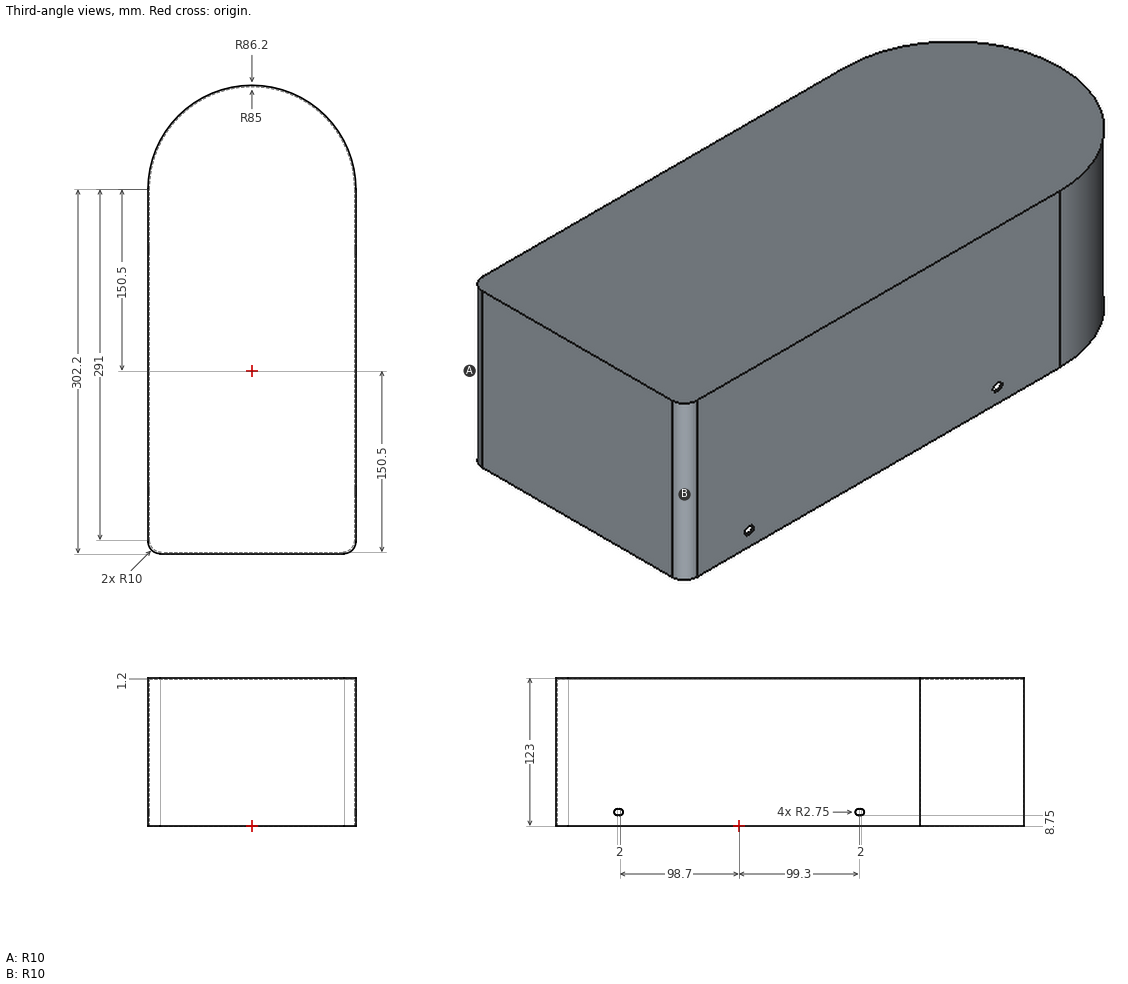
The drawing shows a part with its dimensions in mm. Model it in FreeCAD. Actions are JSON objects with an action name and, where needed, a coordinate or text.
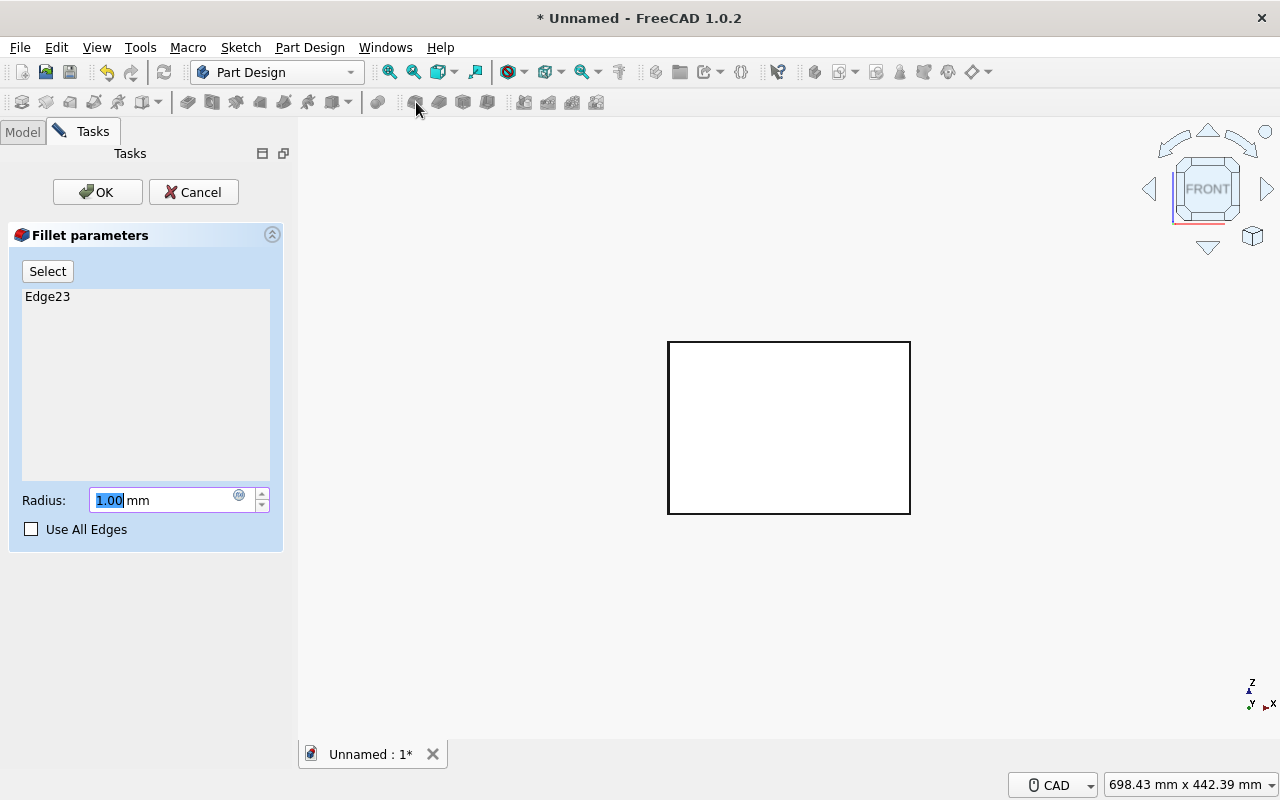
{"action": "type", "text": "10"}
{"action": "key", "text": "Tab"}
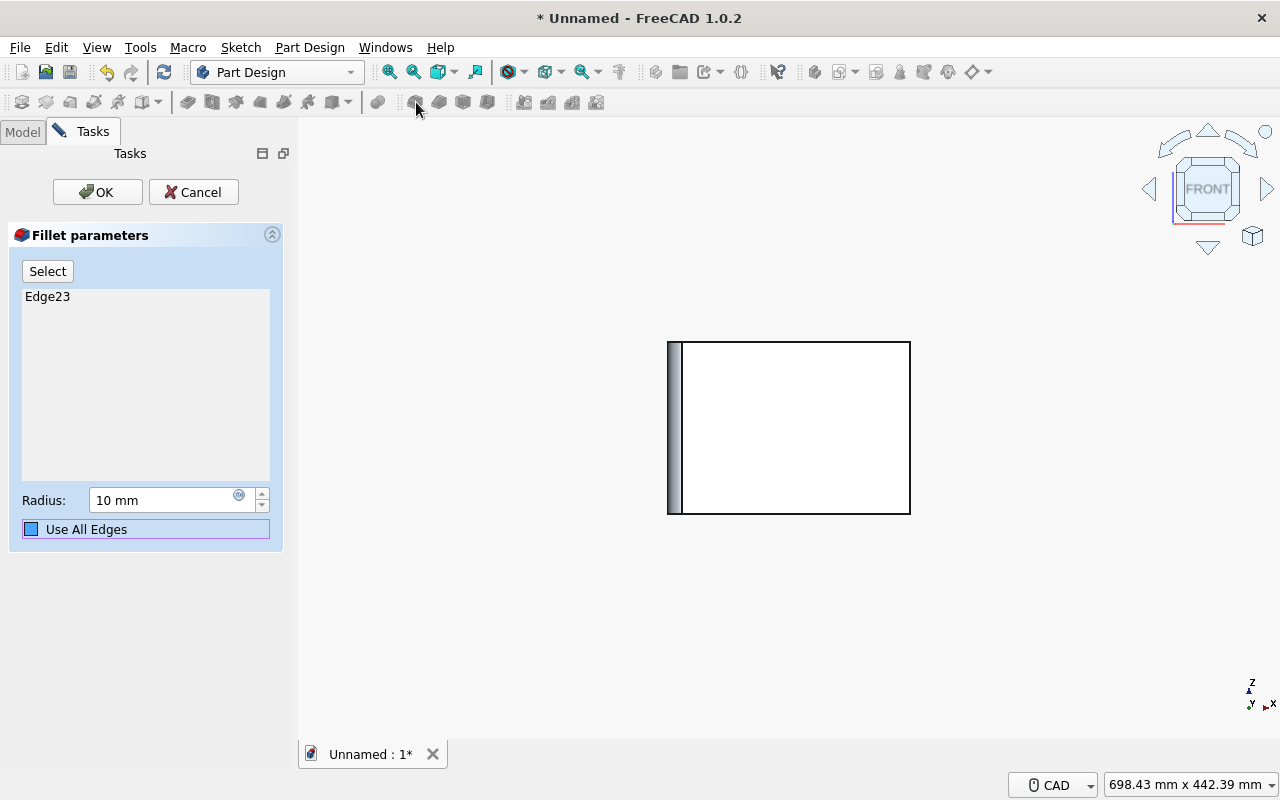
{"action": "left_click", "coordinate": [98, 192]}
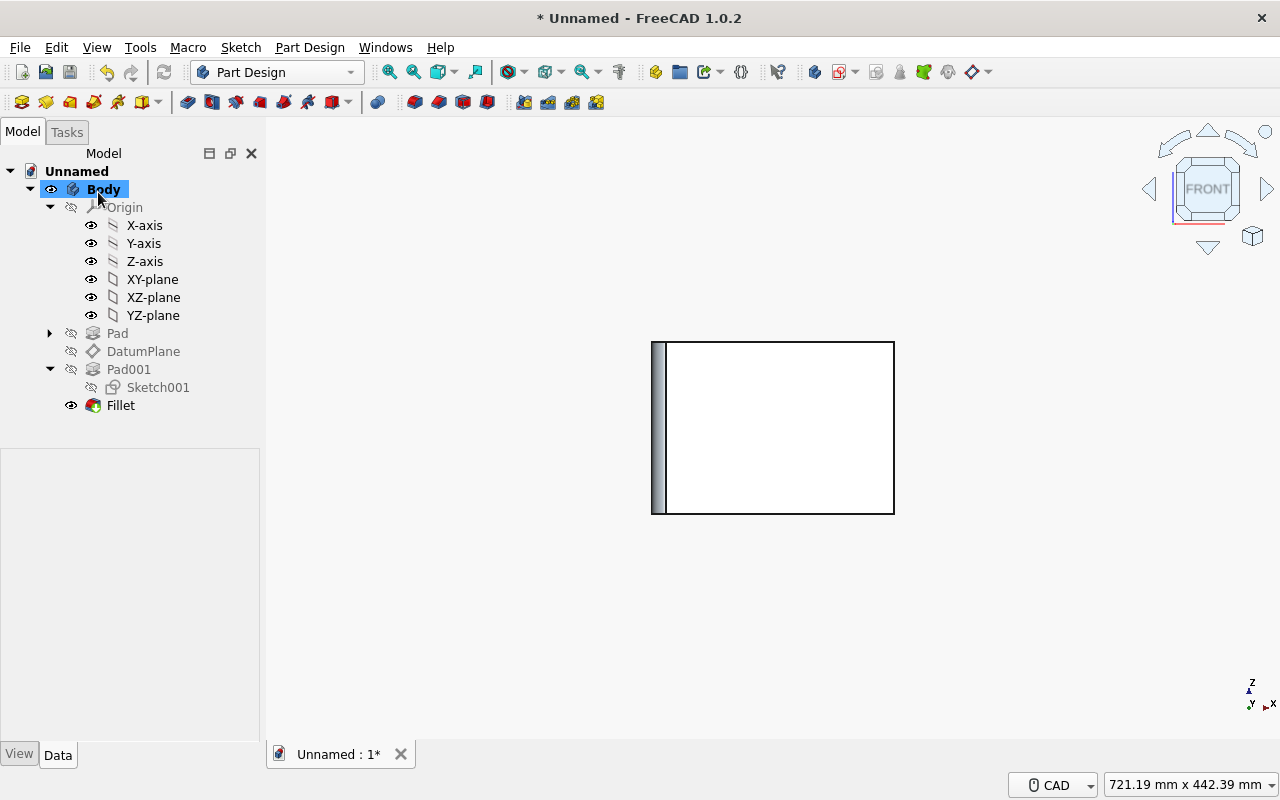
{"action": "key", "text": "v f"}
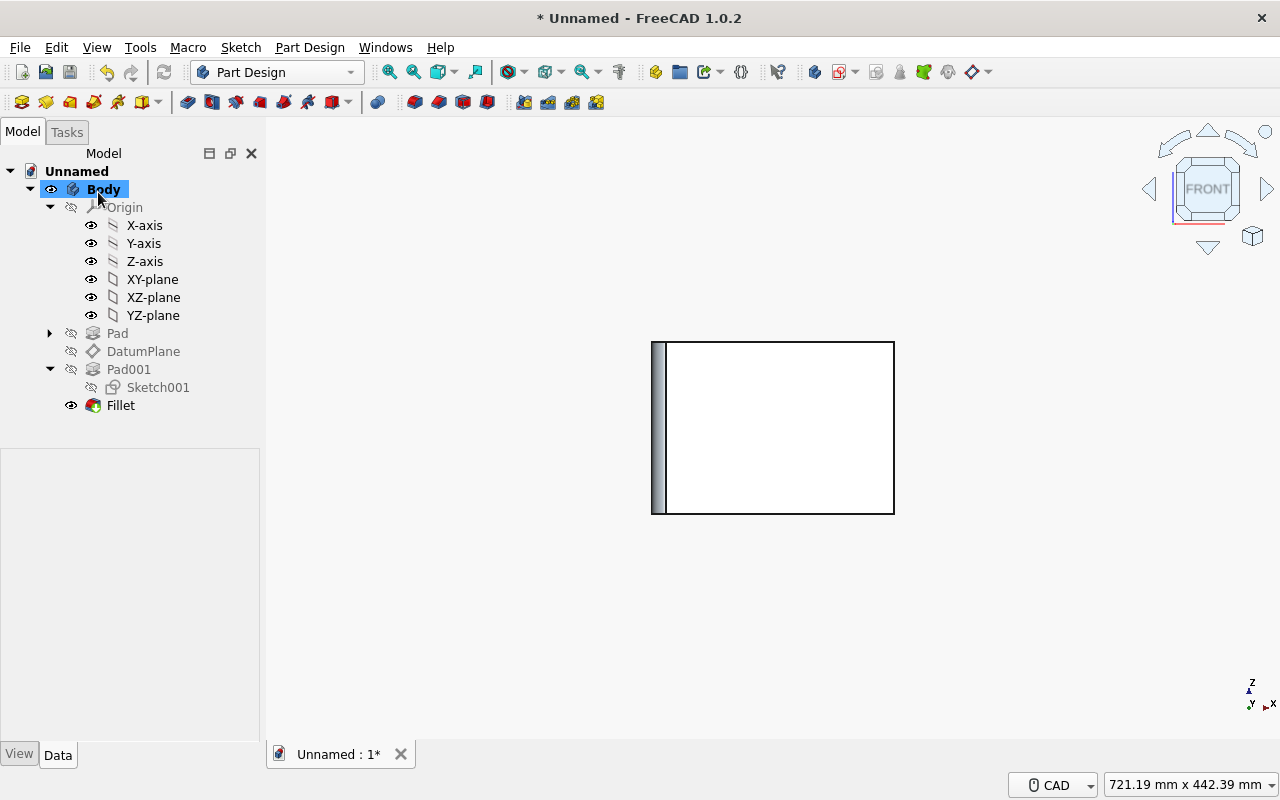
{"action": "left_click", "coordinate": [894, 427]}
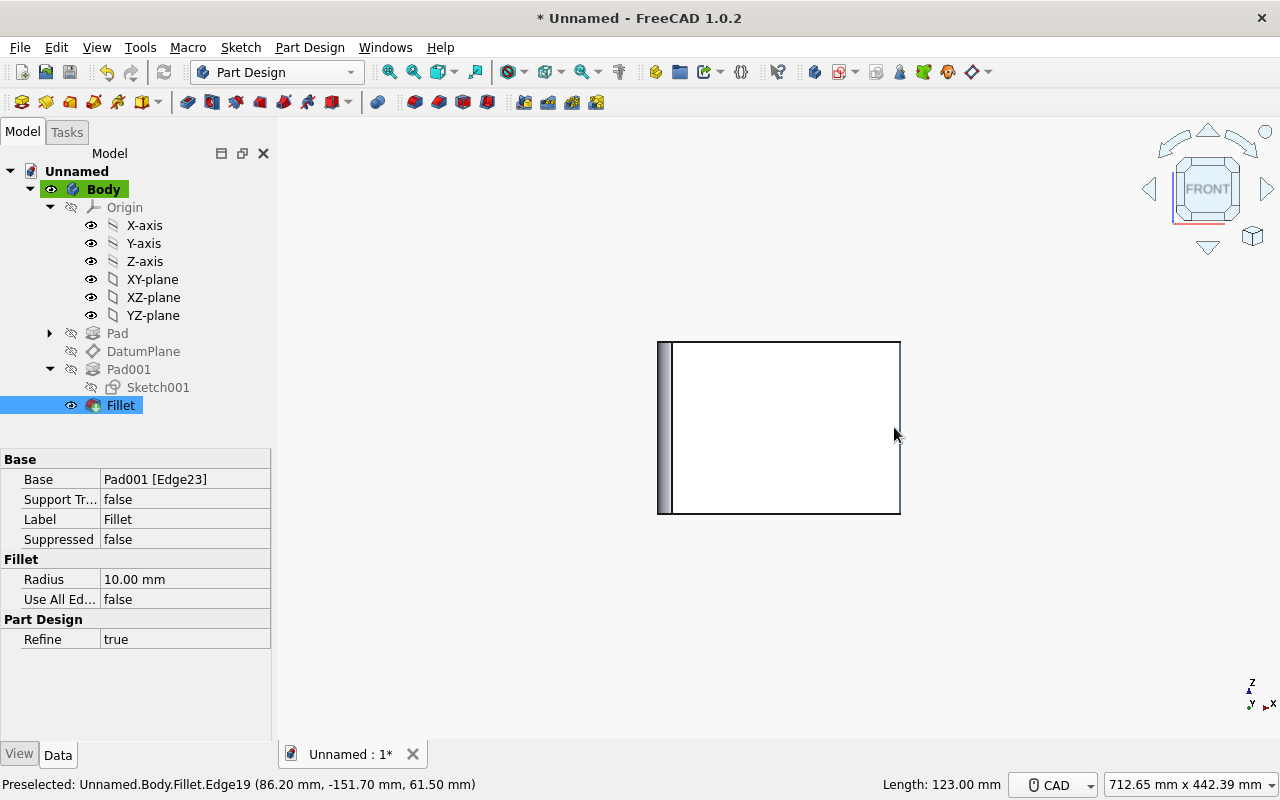
{"action": "left_click", "coordinate": [416, 102]}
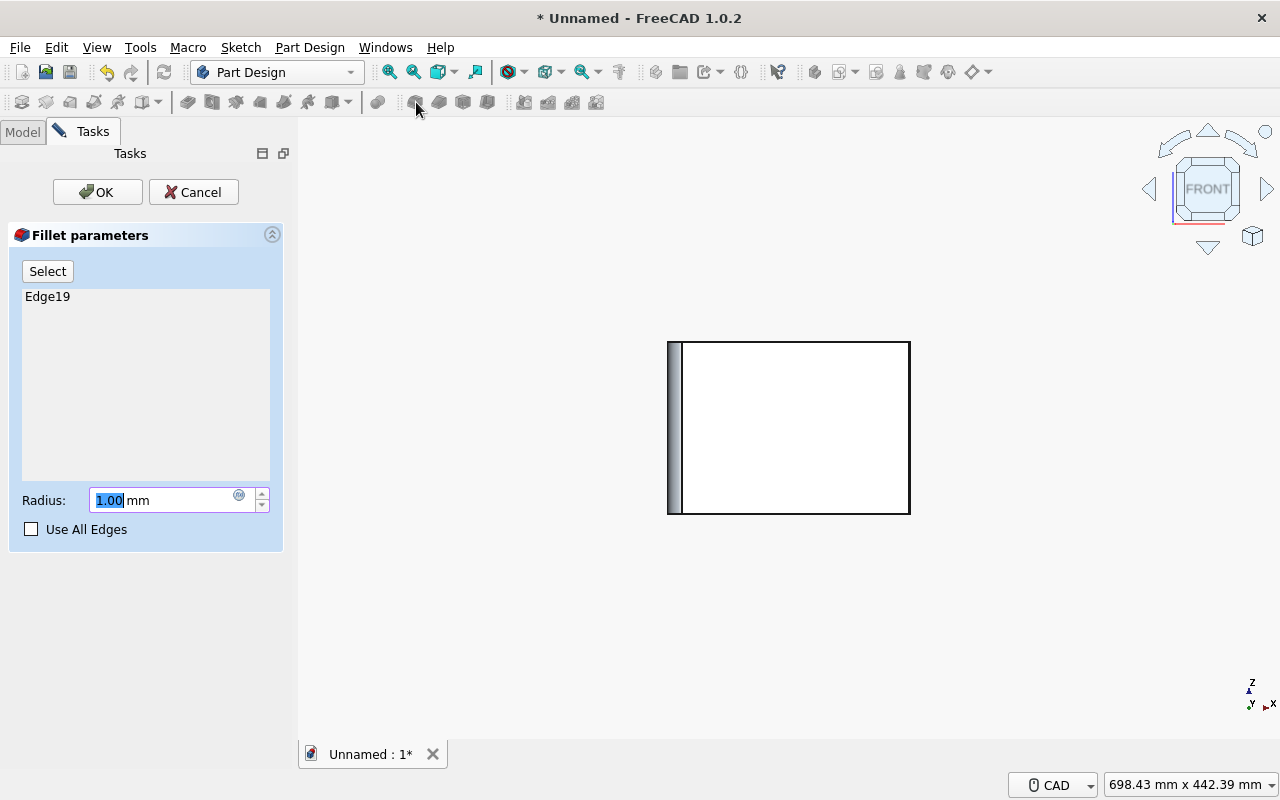
{"action": "type", "text": "10"}
{"action": "key", "text": "Tab"}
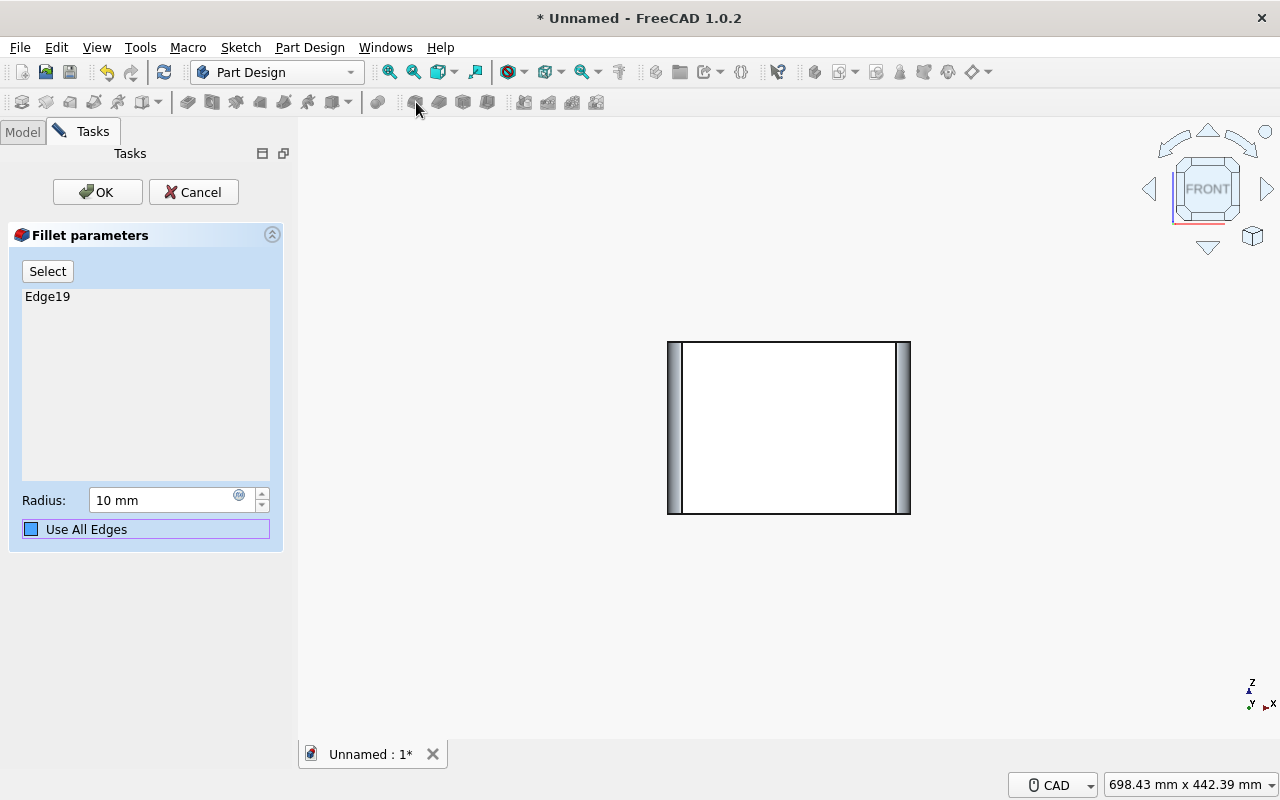
{"action": "left_click", "coordinate": [98, 192]}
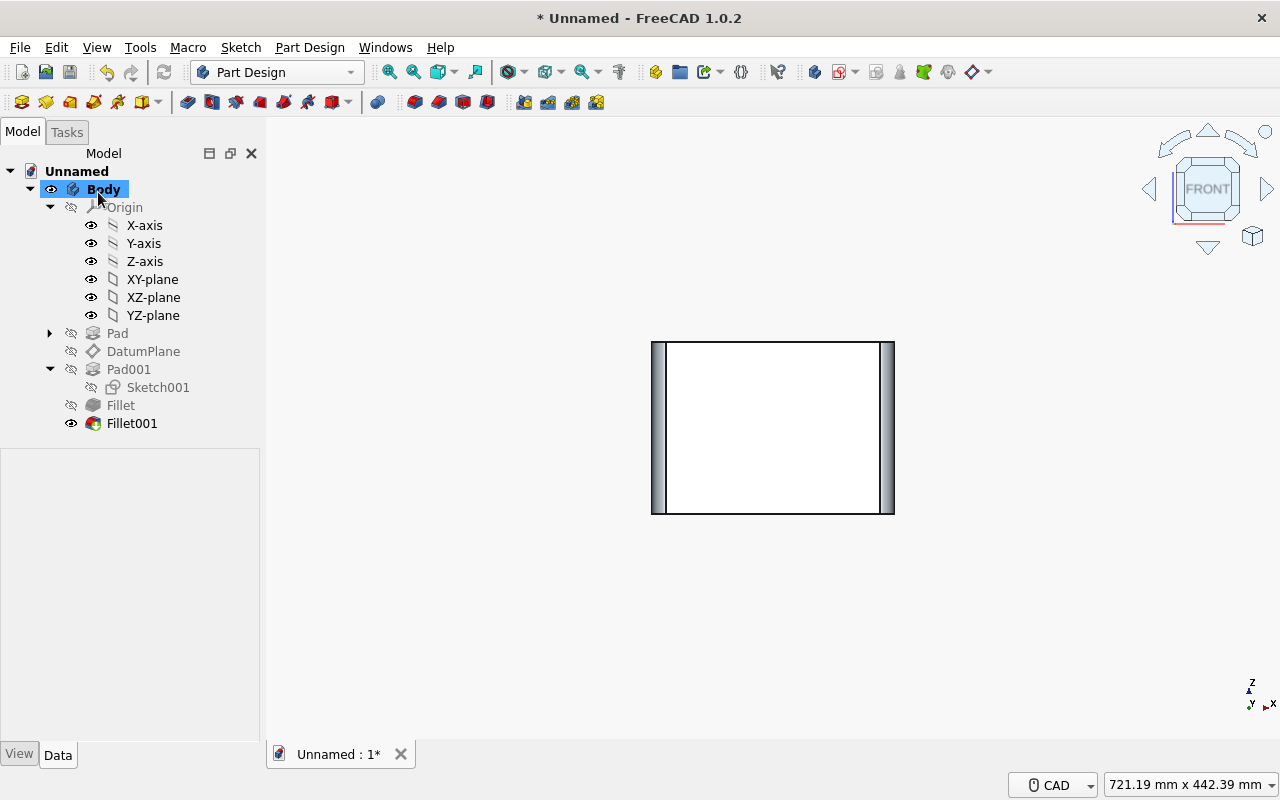
{"action": "left_click", "coordinate": [390, 72]}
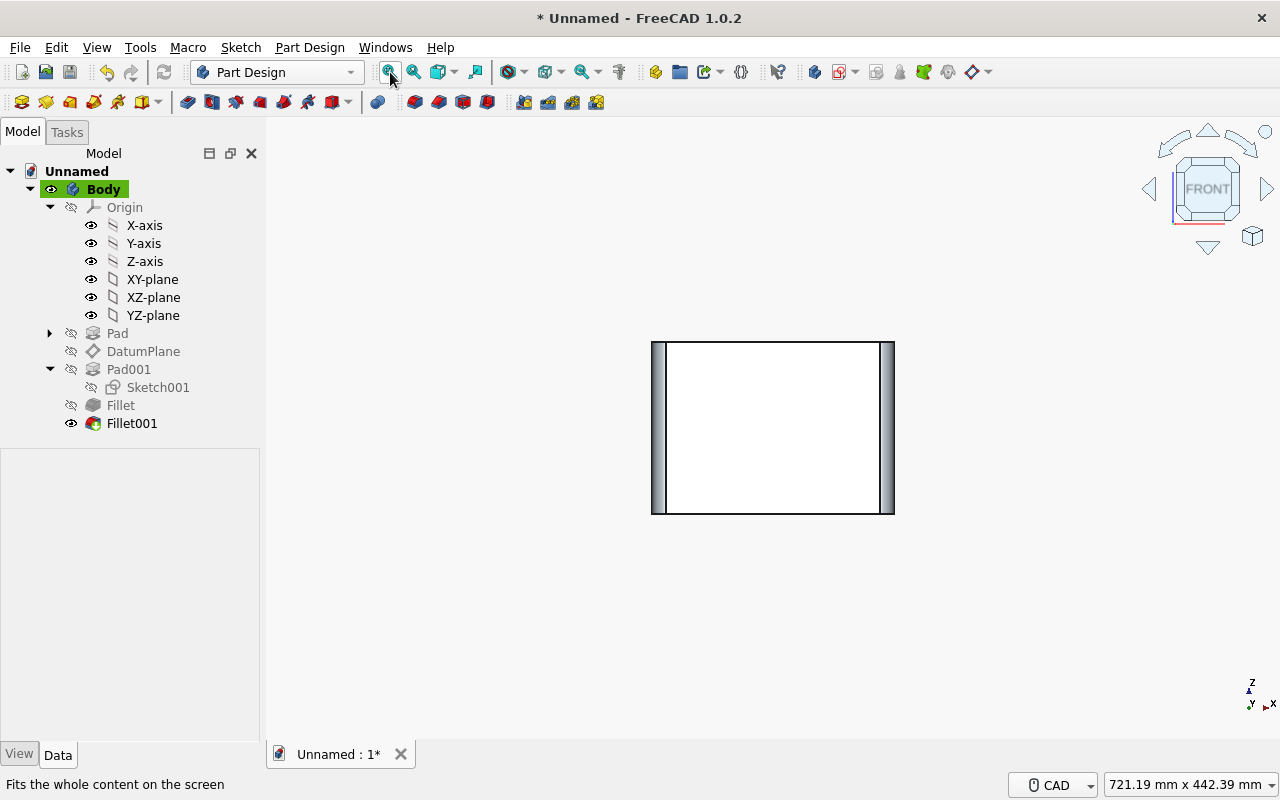
{"action": "key", "text": "6"}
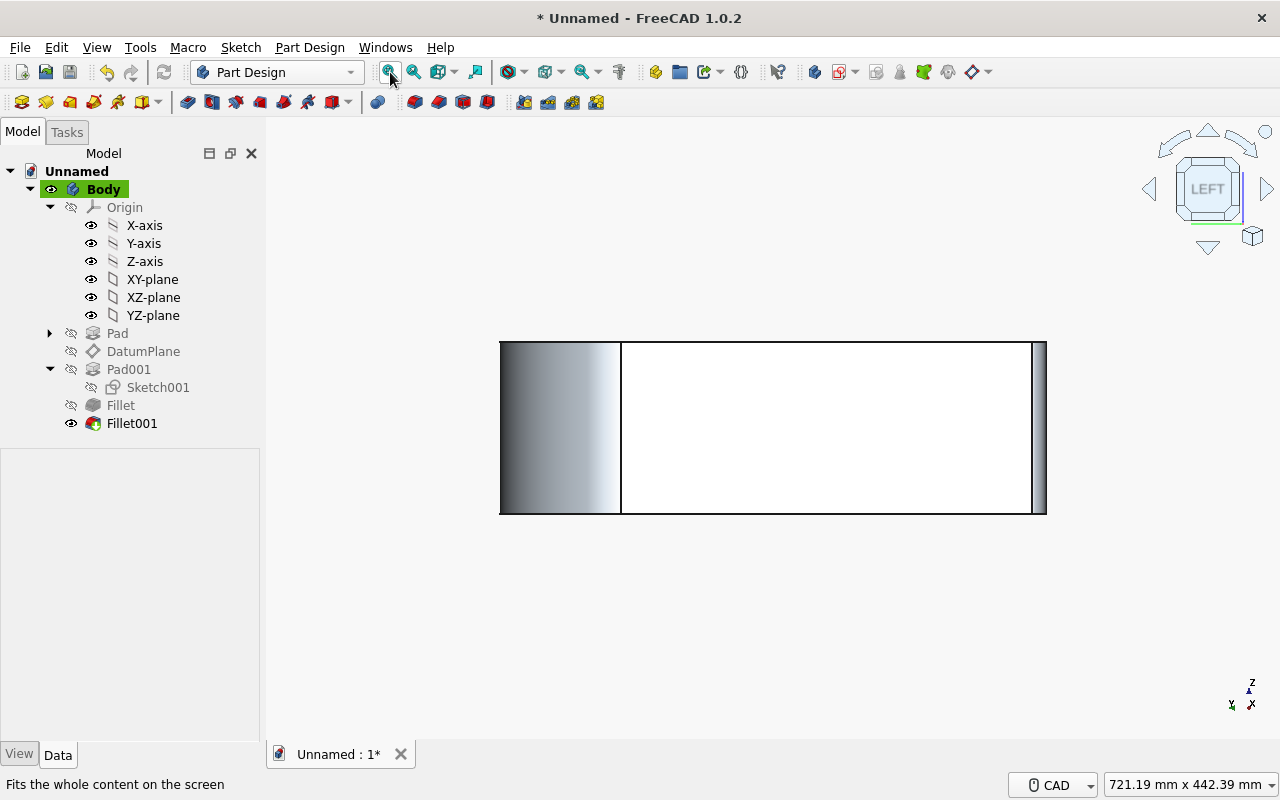
{"action": "left_click", "coordinate": [709, 427]}